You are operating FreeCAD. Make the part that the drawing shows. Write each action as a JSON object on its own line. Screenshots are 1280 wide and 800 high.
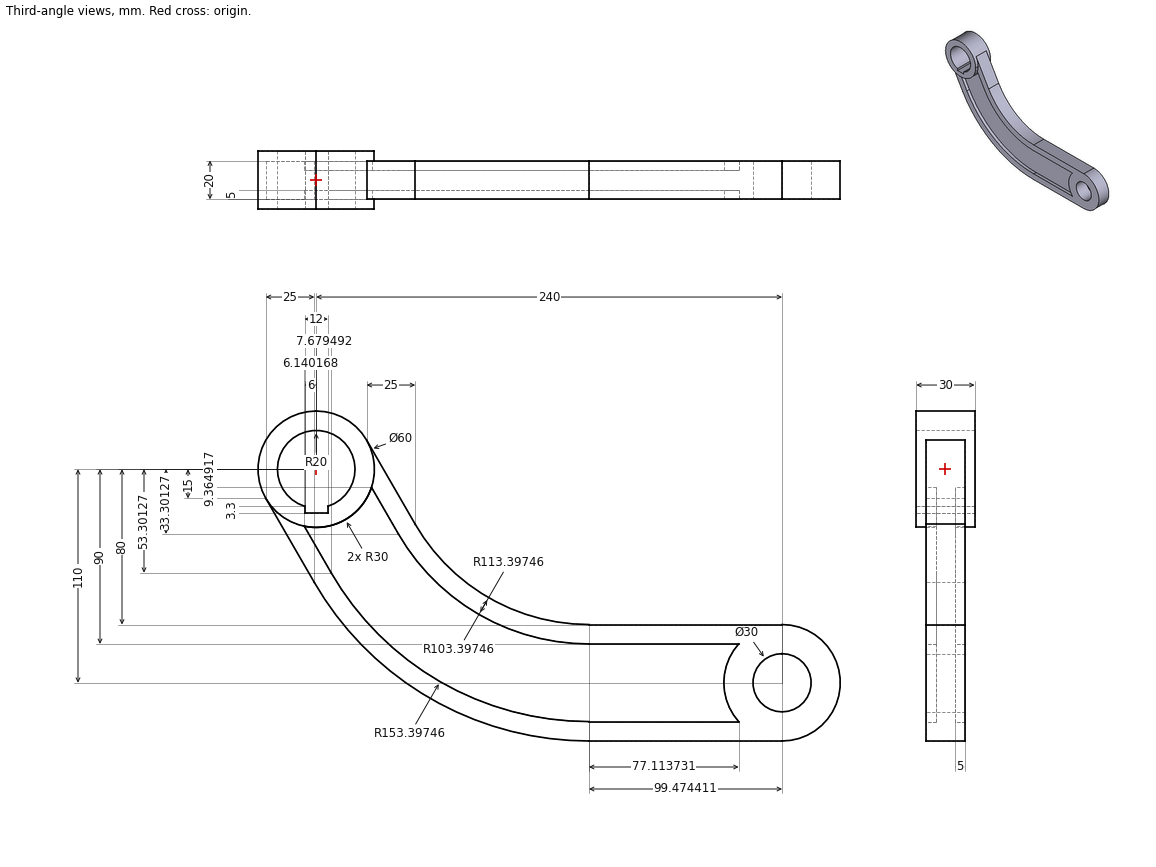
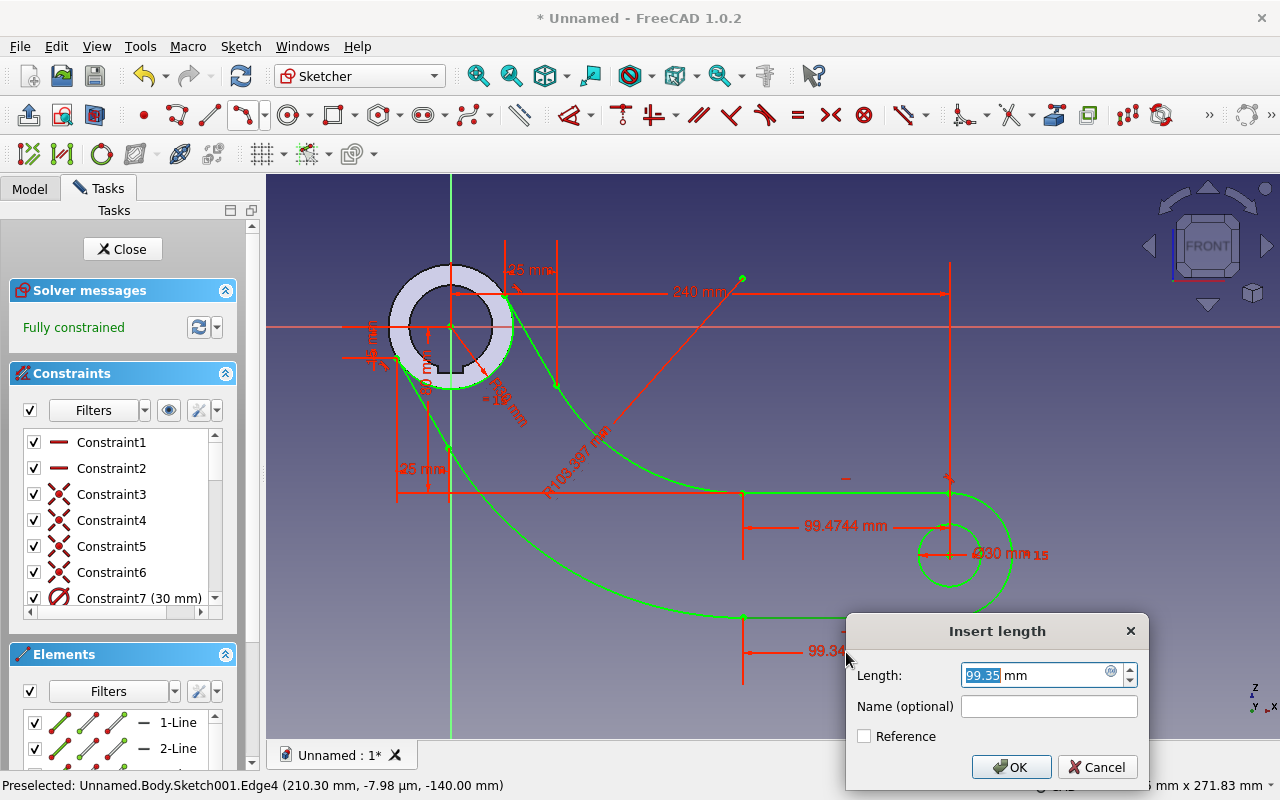
{"action": "type", "text": "99.474411"}
{"action": "key", "text": "Return"}
{"action": "key", "text": "Escape"}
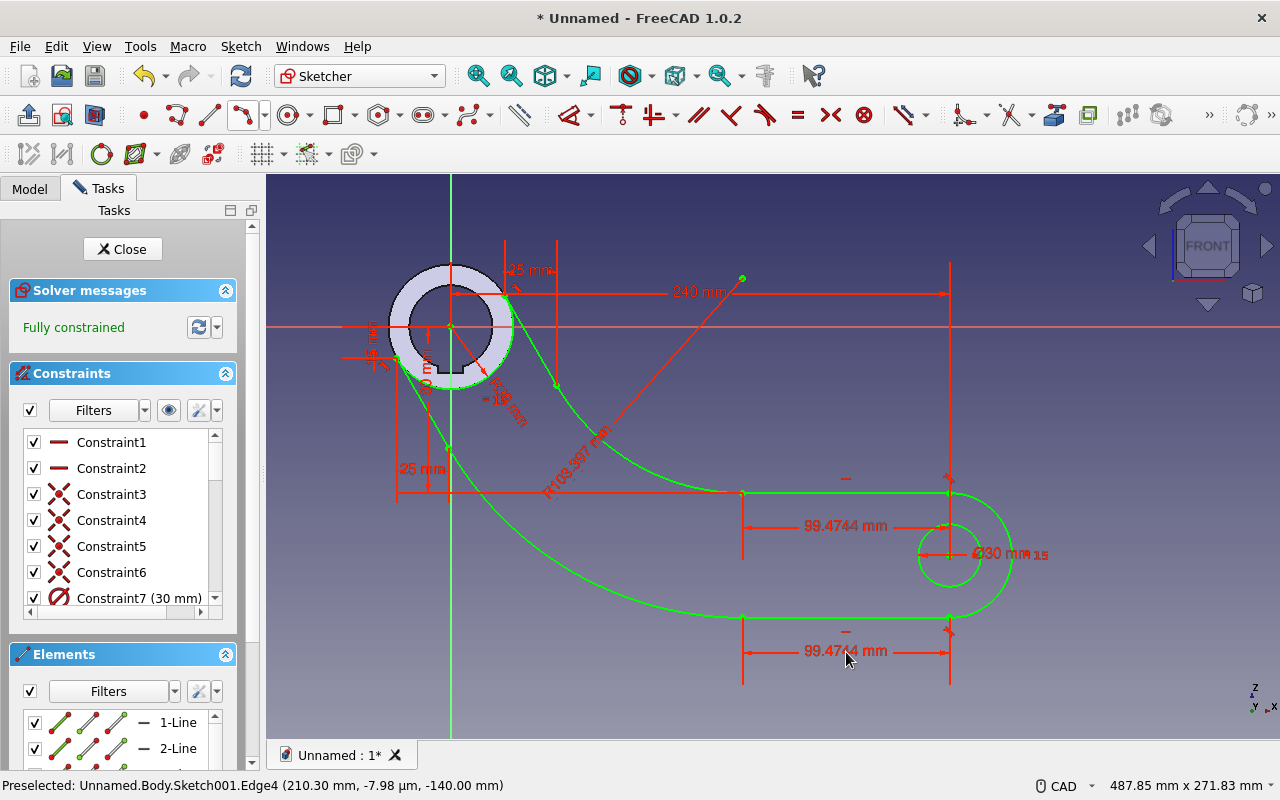
{"action": "left_click", "coordinate": [123, 249]}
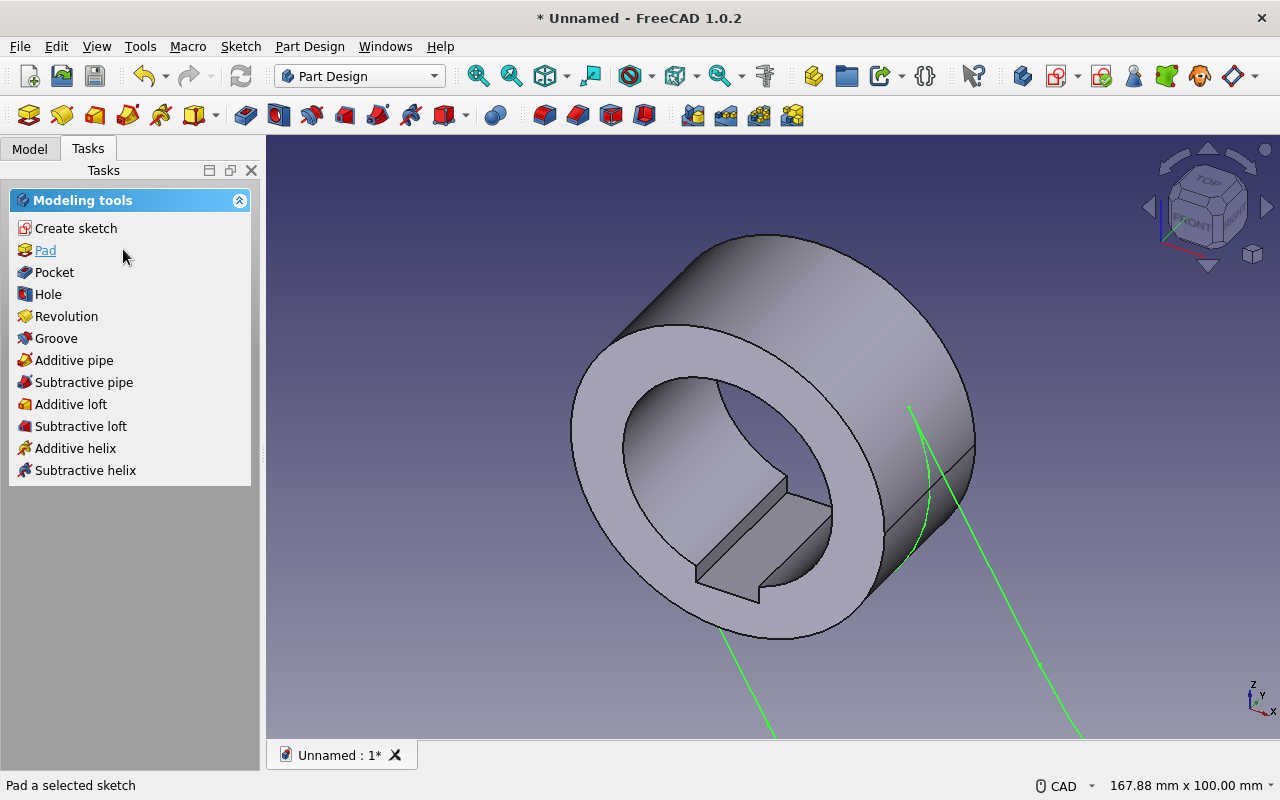
{"action": "left_click", "coordinate": [29, 116]}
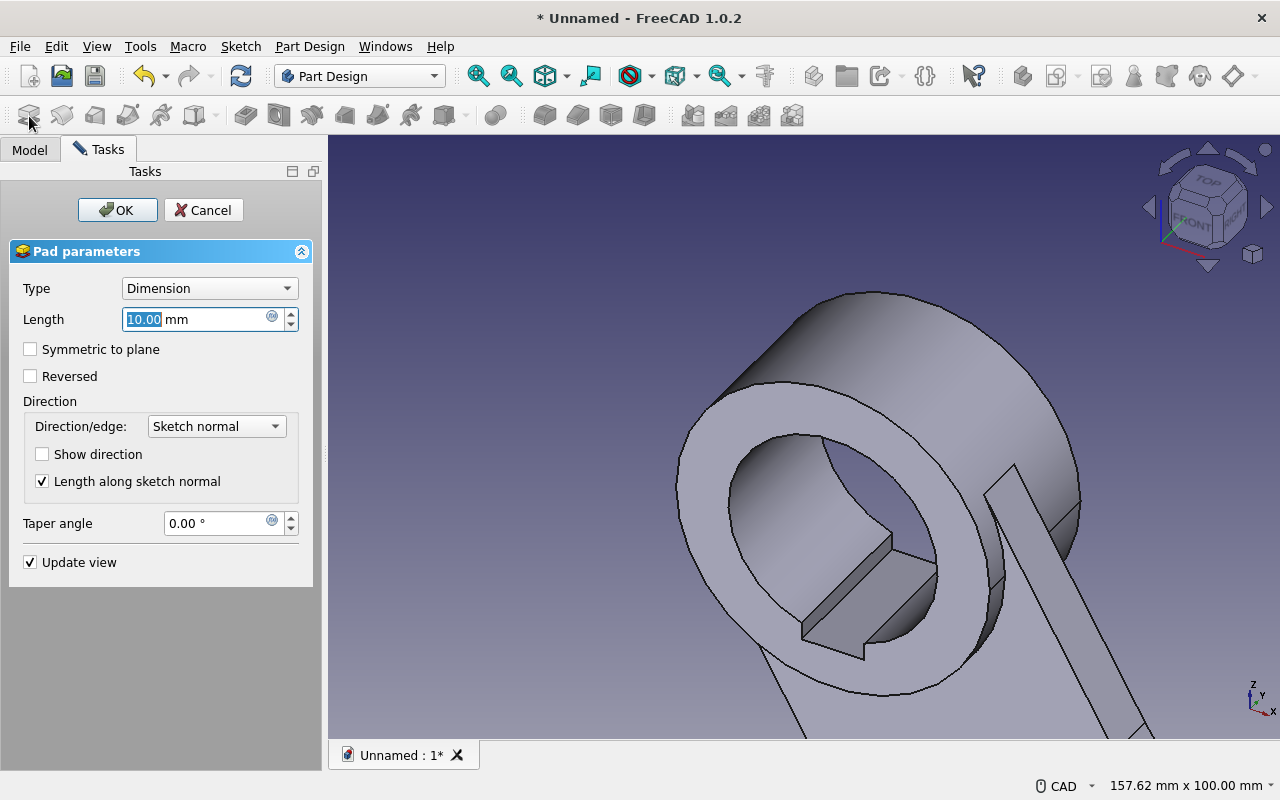
{"action": "type", "text": "20"}
{"action": "key", "text": "Tab"}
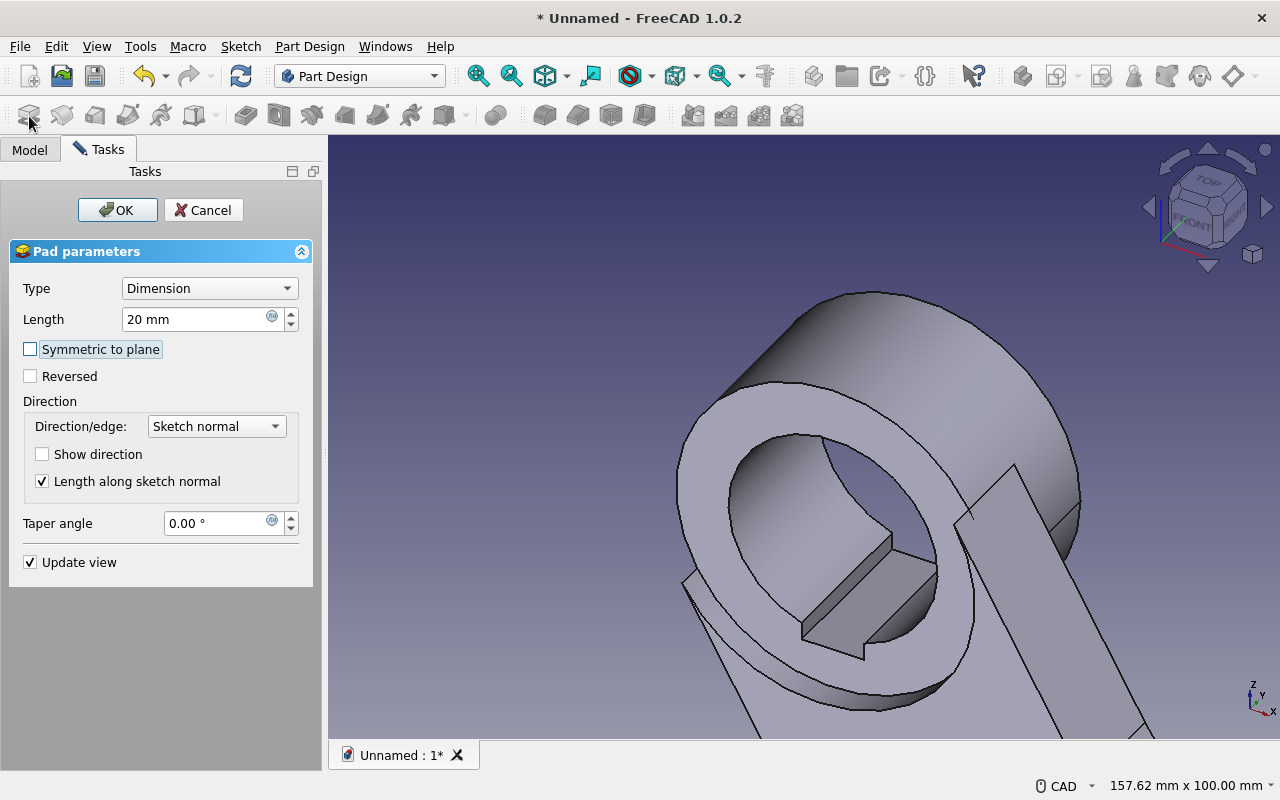
{"action": "left_click", "coordinate": [31, 349]}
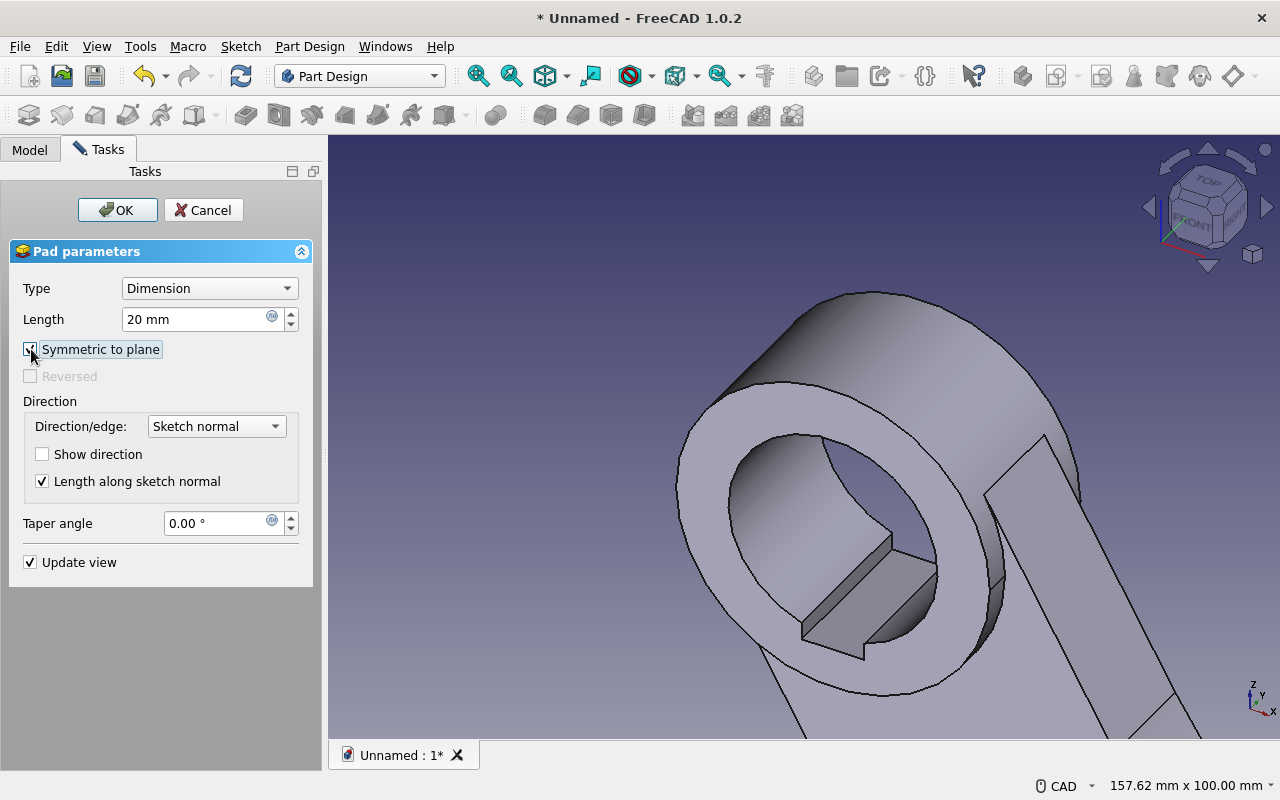
{"action": "left_click", "coordinate": [118, 210]}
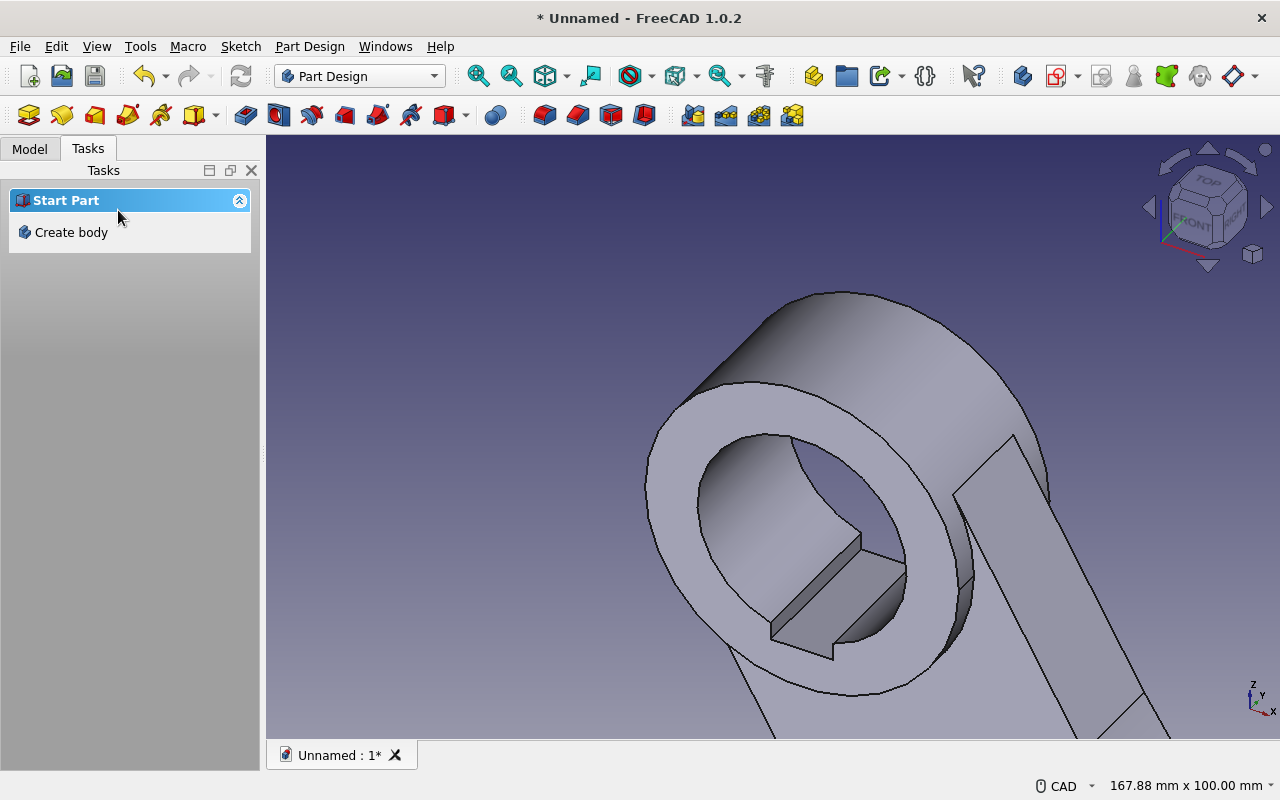
{"action": "left_click", "coordinate": [479, 76]}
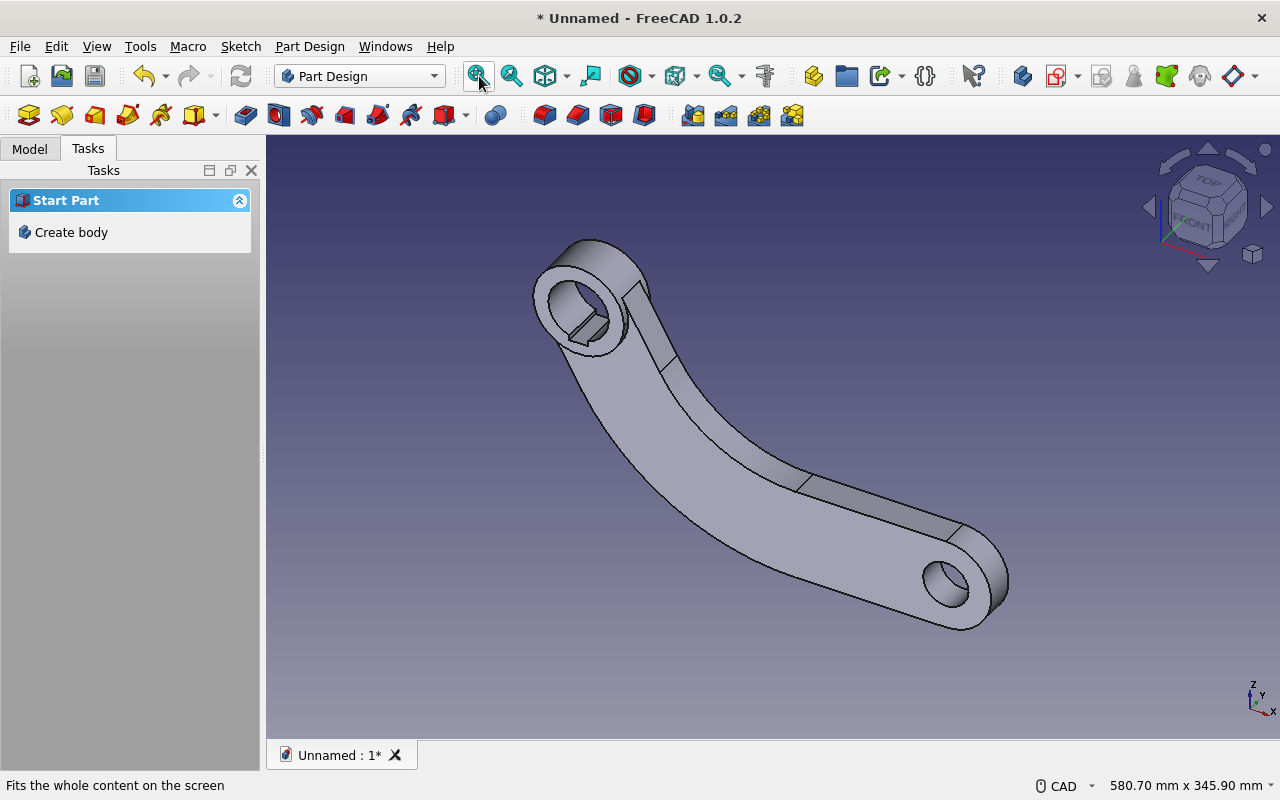
{"action": "key", "text": "4"}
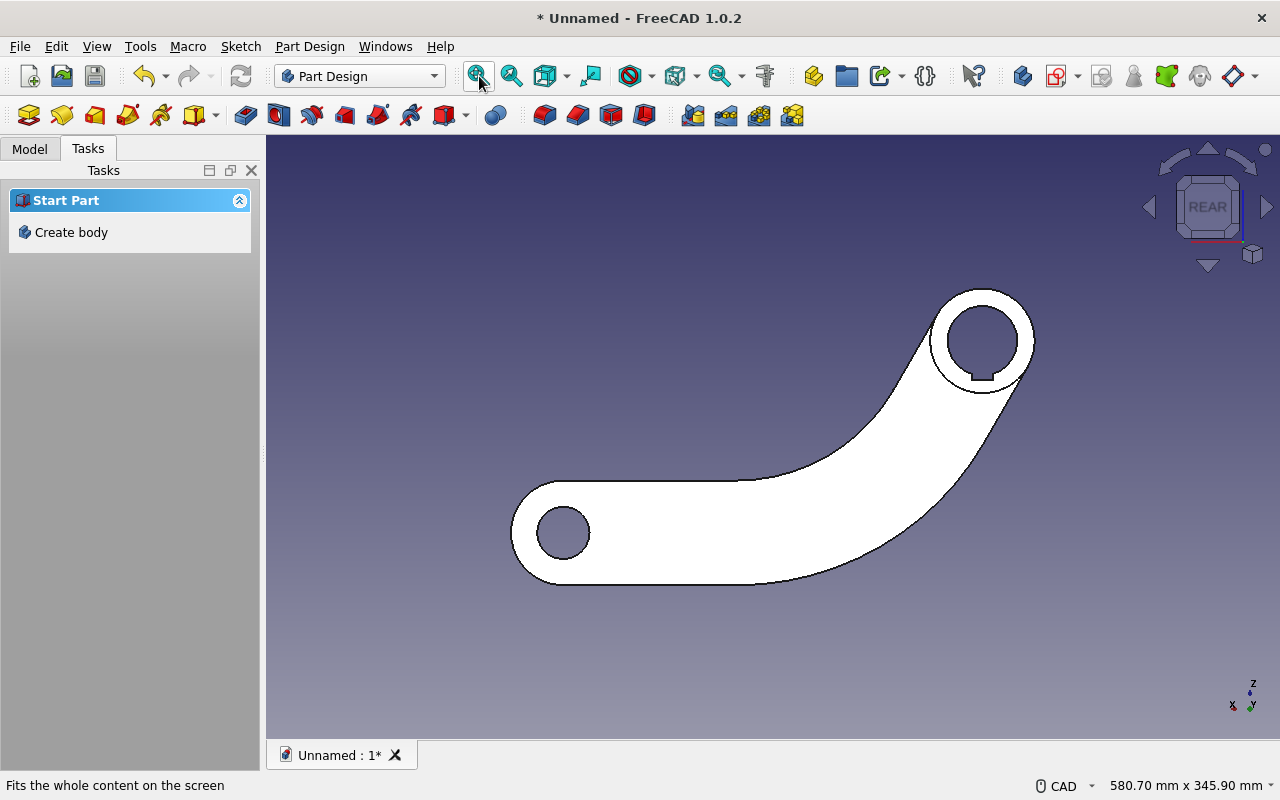
{"action": "left_click", "coordinate": [917, 449]}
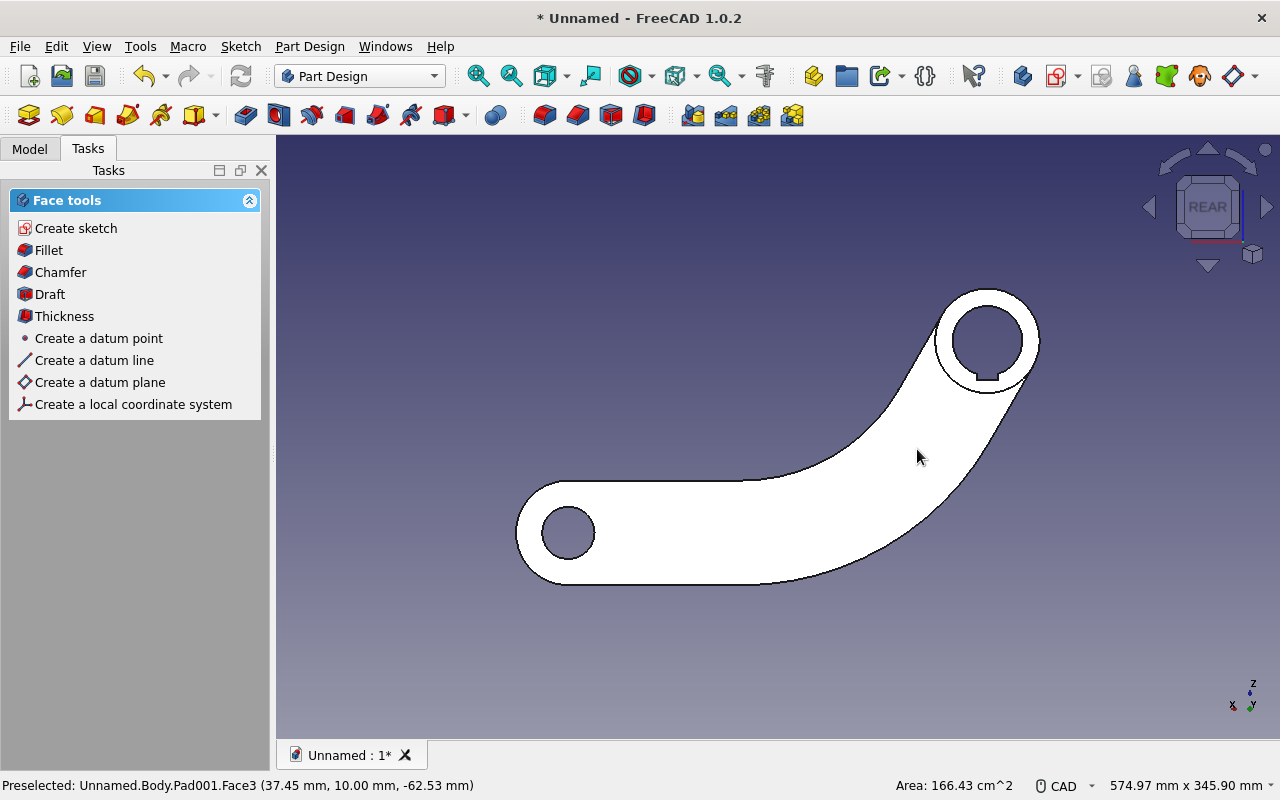
{"action": "left_click", "coordinate": [1056, 76]}